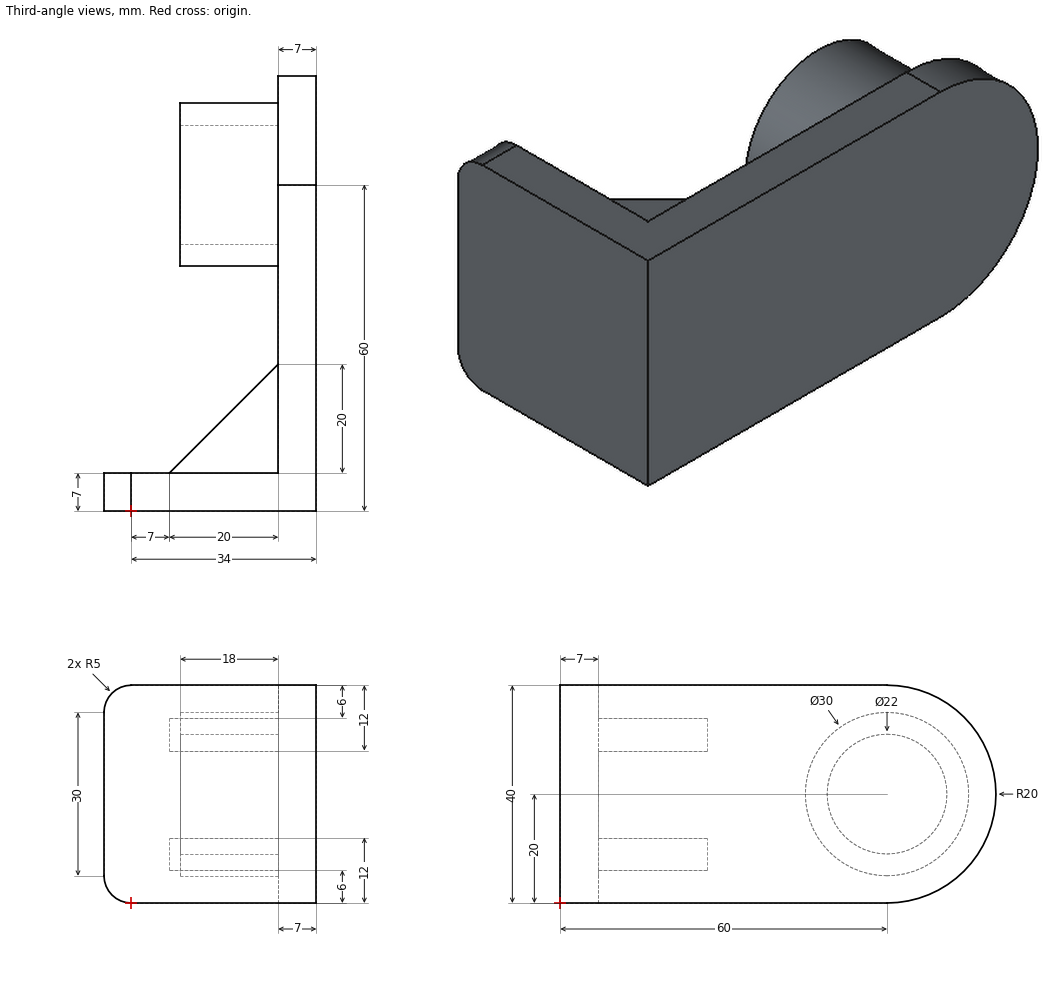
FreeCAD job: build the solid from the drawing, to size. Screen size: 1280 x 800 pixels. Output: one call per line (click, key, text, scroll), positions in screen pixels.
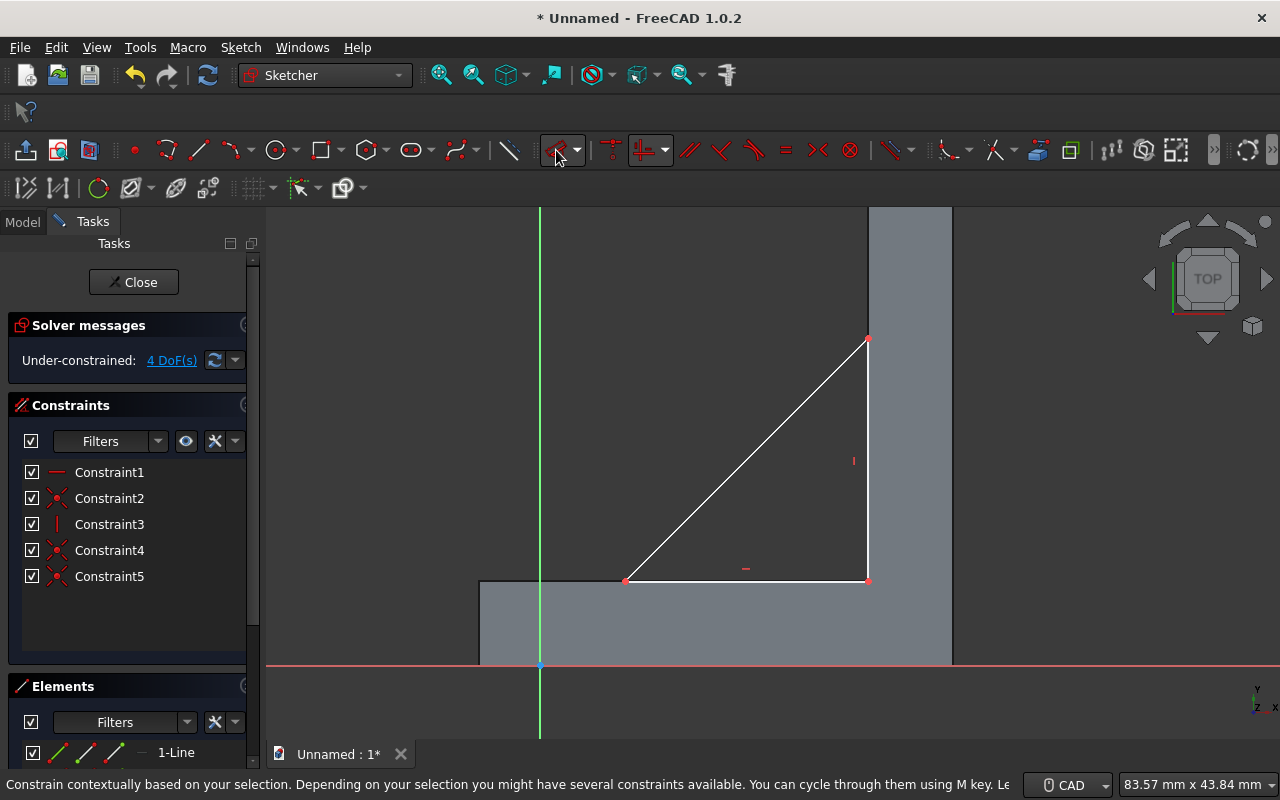
click(698, 582)
click(747, 616)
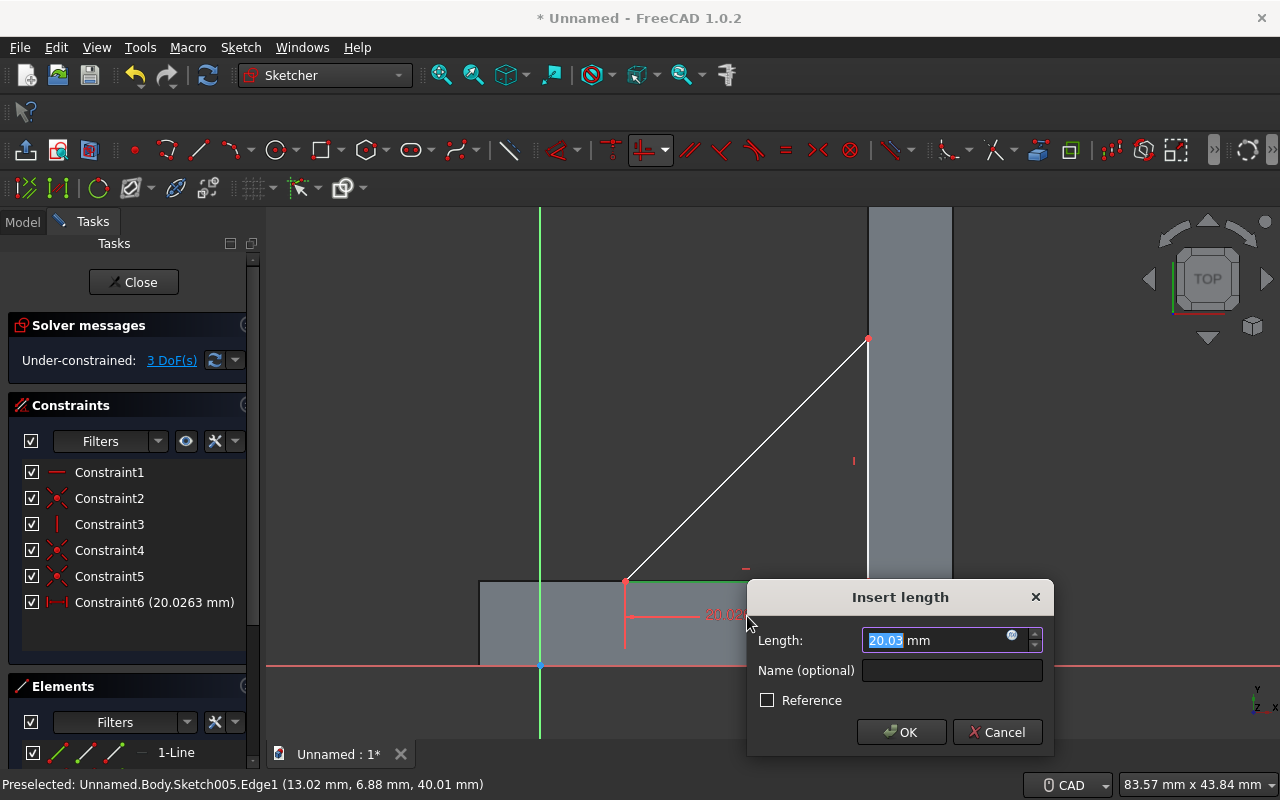
text(20)
key(Return)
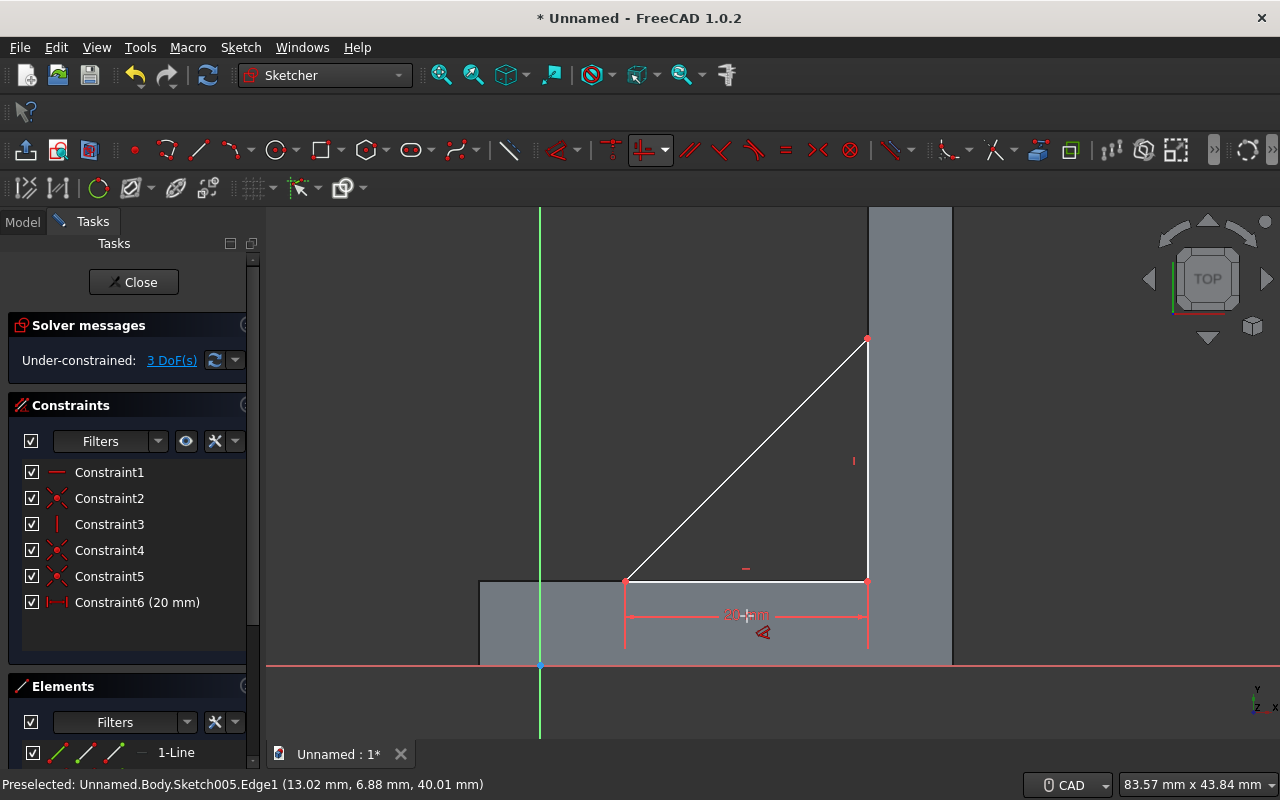
click(868, 509)
click(902, 461)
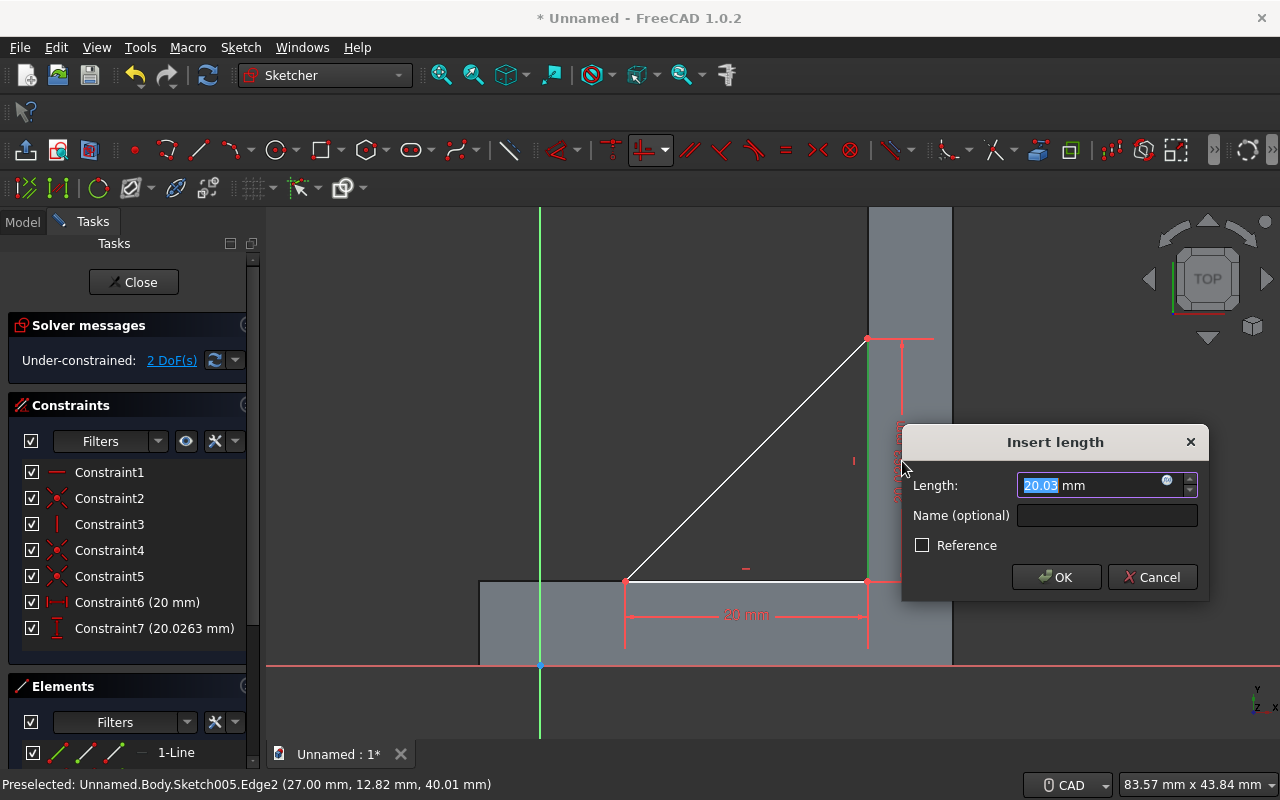
text(20)
key(Return)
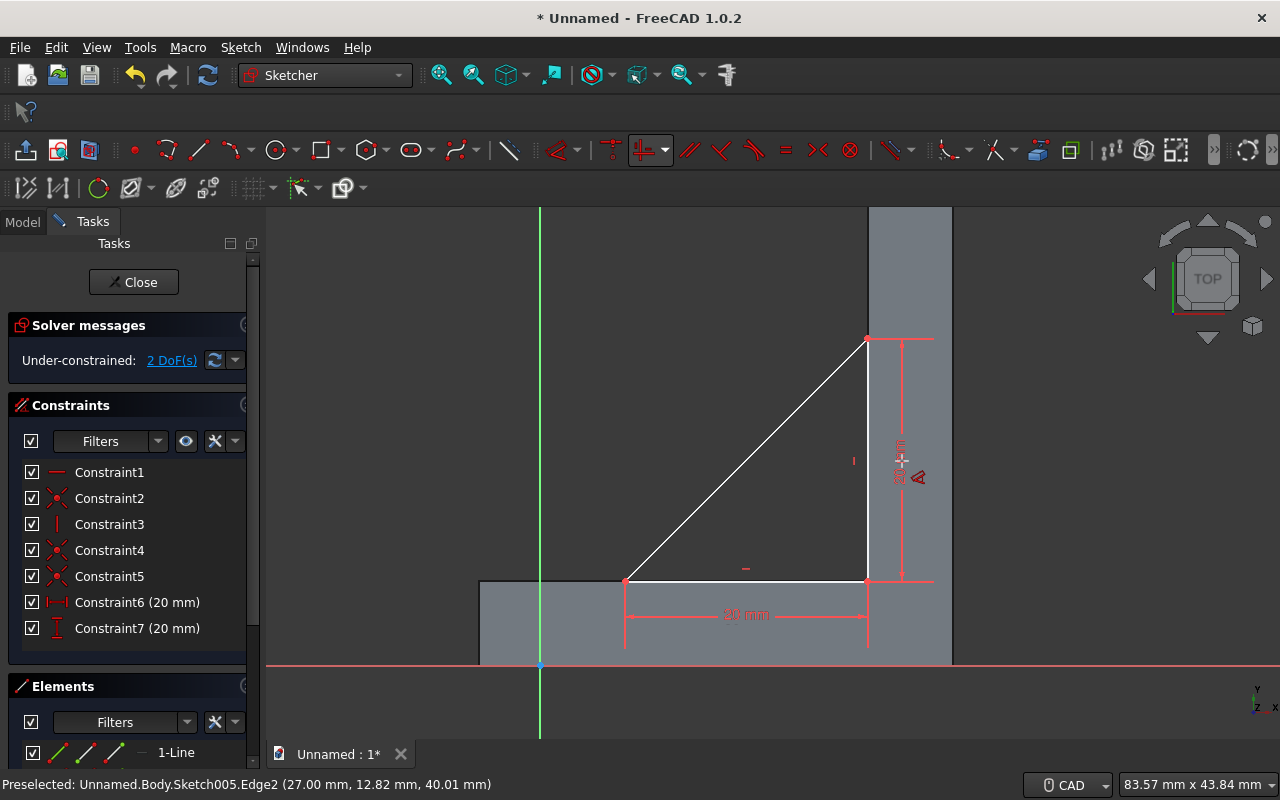
click(625, 582)
click(583, 700)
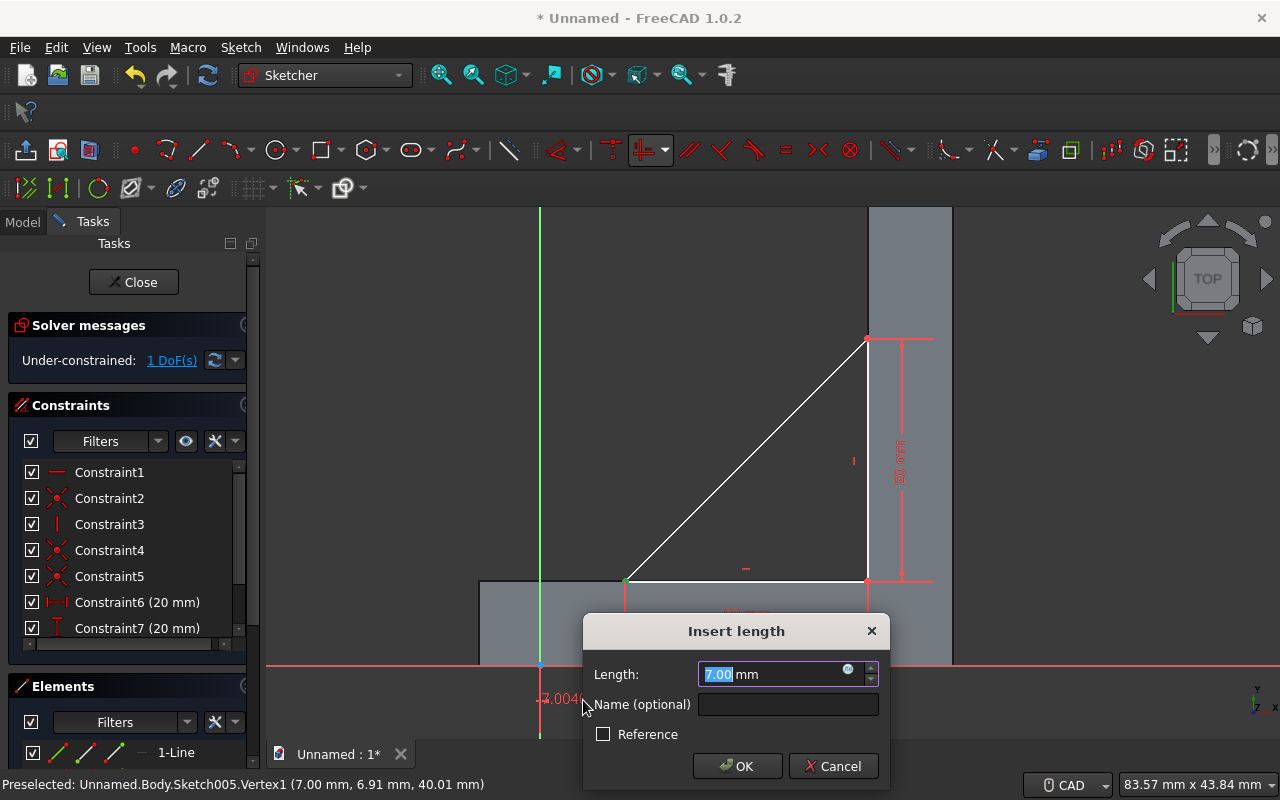
text(7)
key(Return)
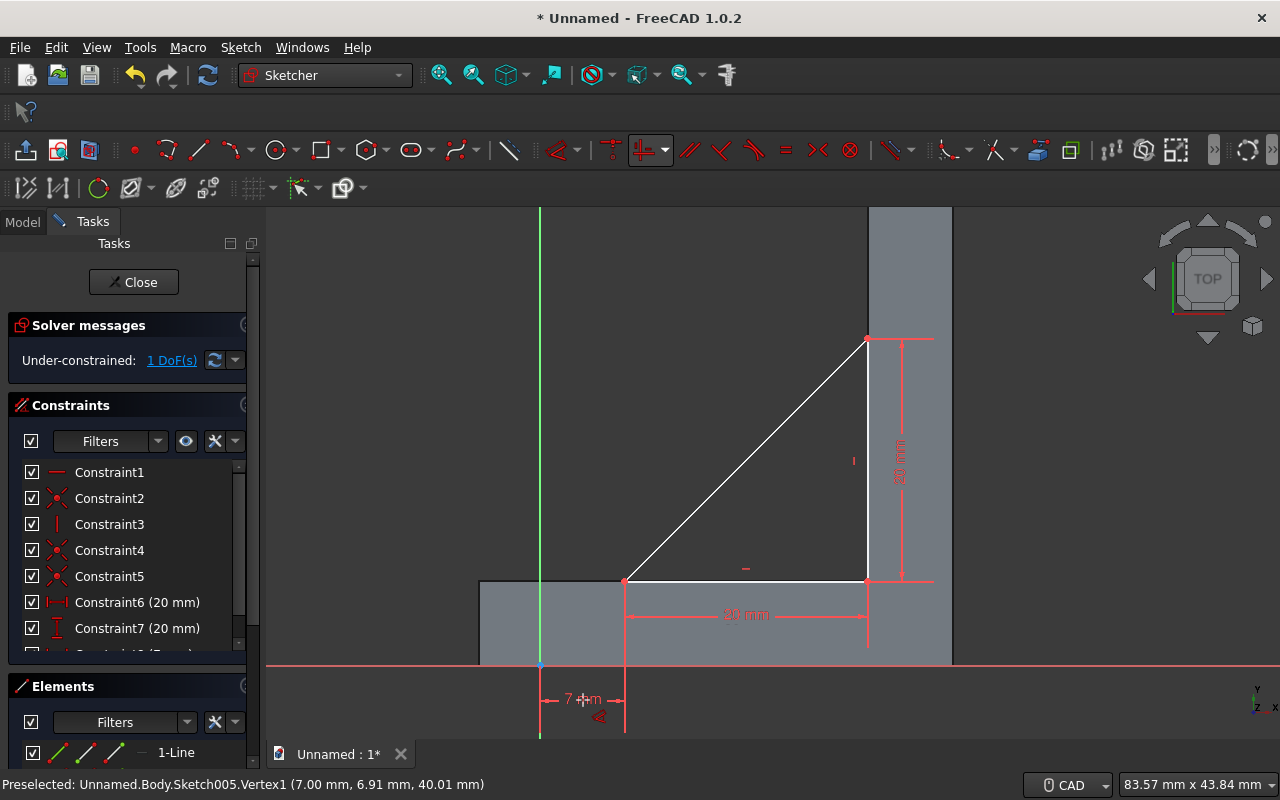
click(625, 582)
click(506, 624)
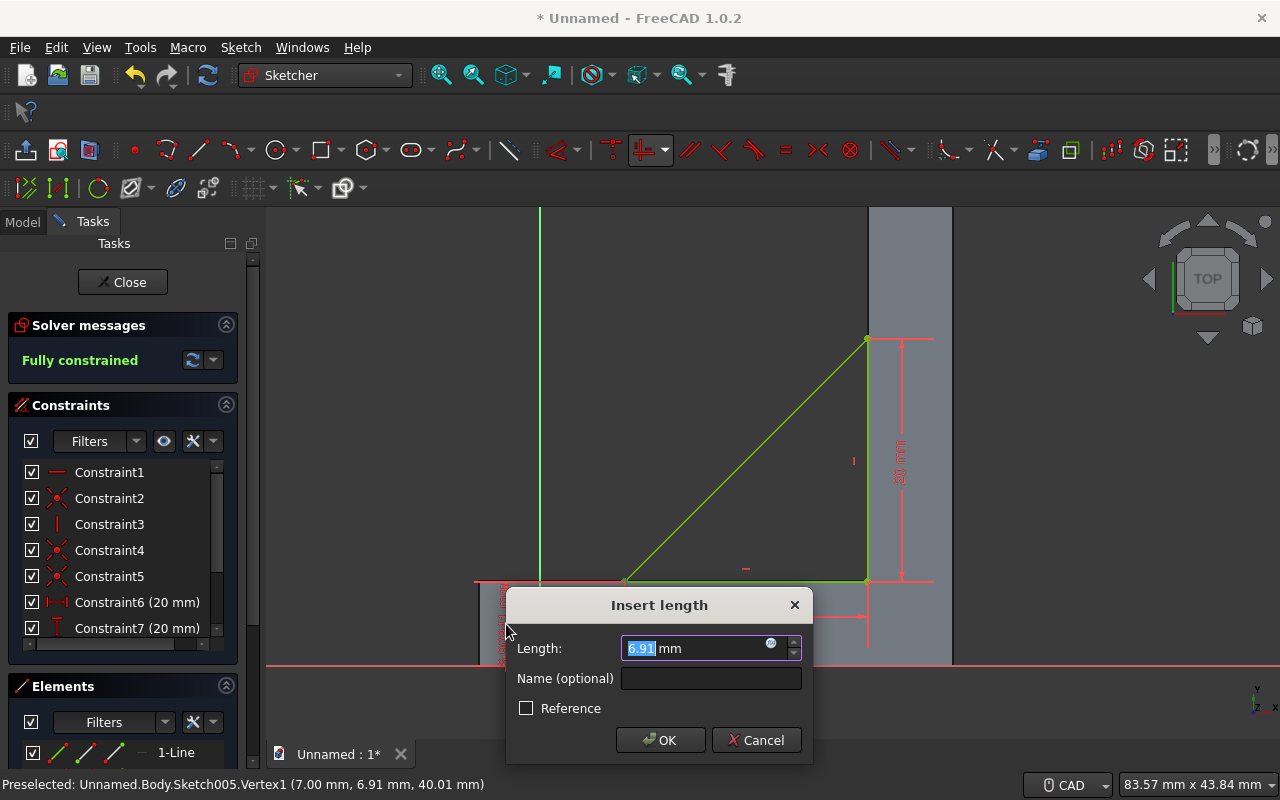
text(7)
key(Return)
key(Escape)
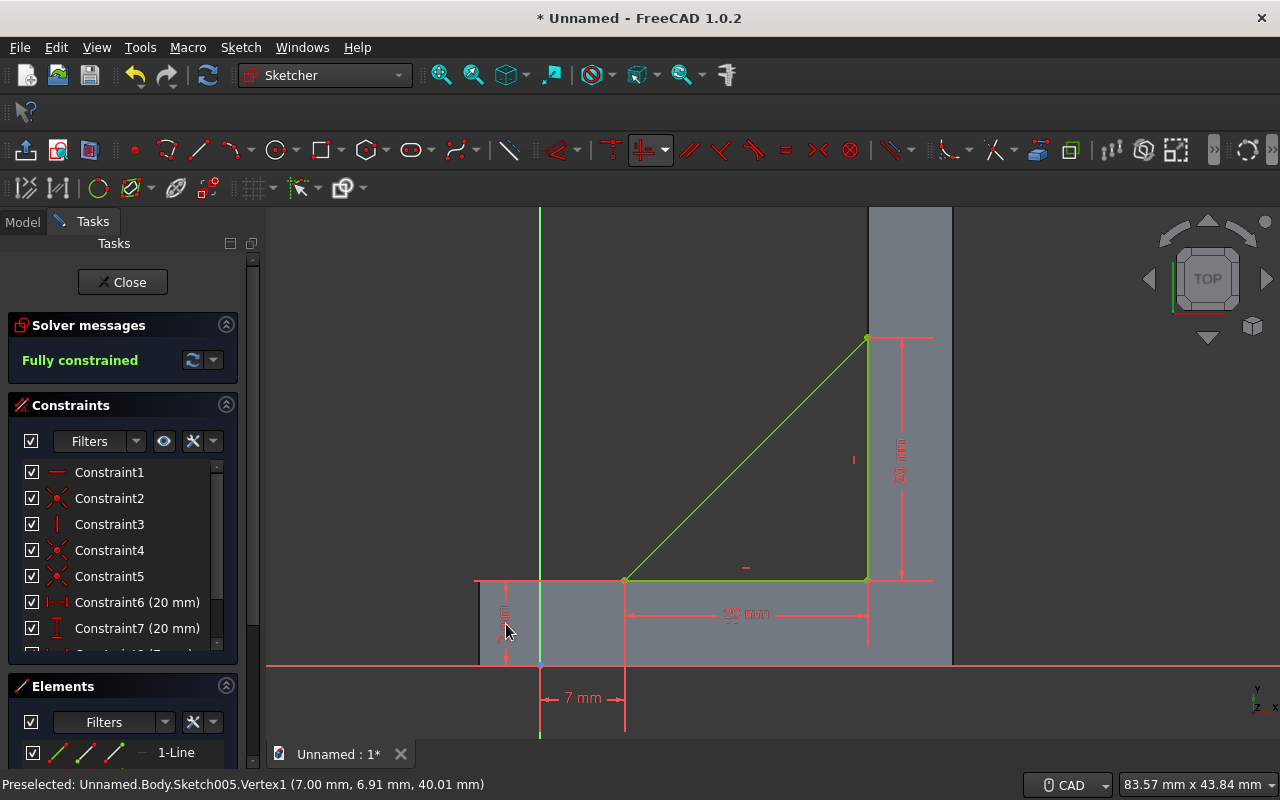
click(123, 282)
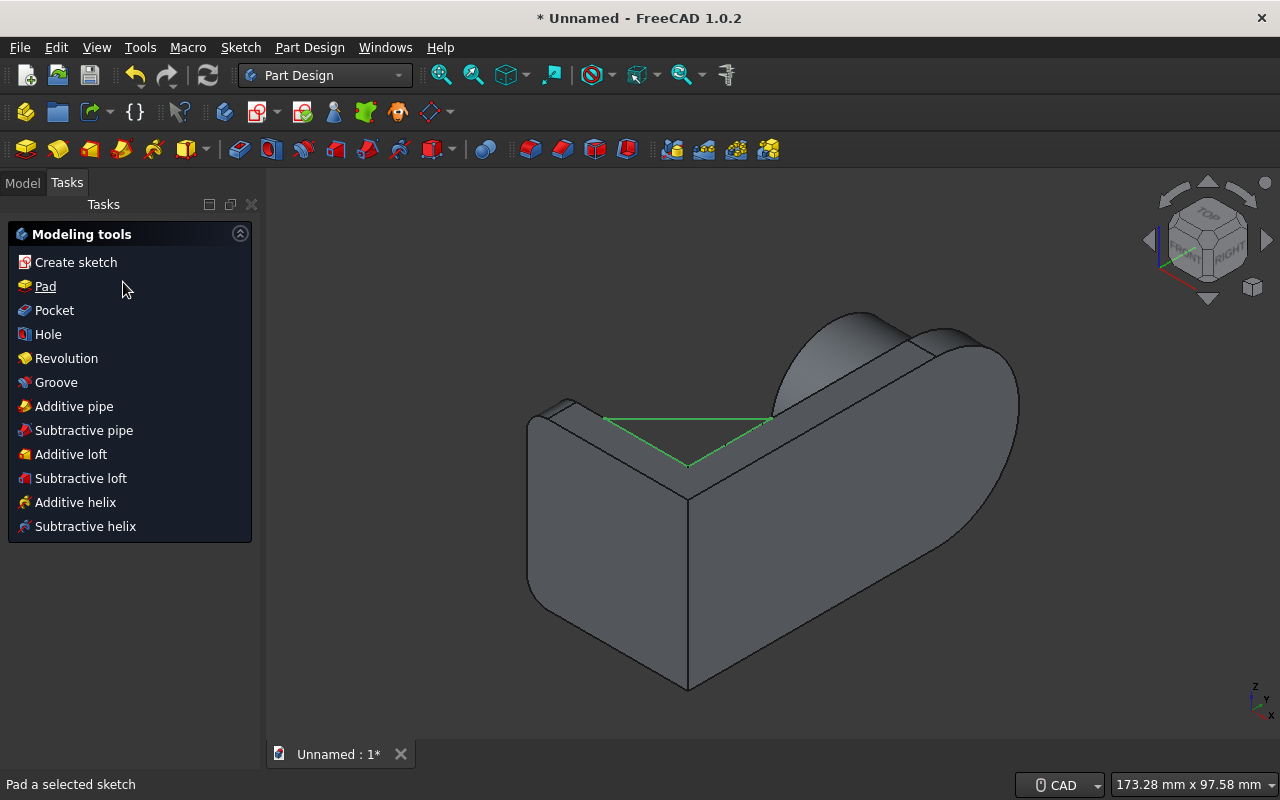
click(26, 150)